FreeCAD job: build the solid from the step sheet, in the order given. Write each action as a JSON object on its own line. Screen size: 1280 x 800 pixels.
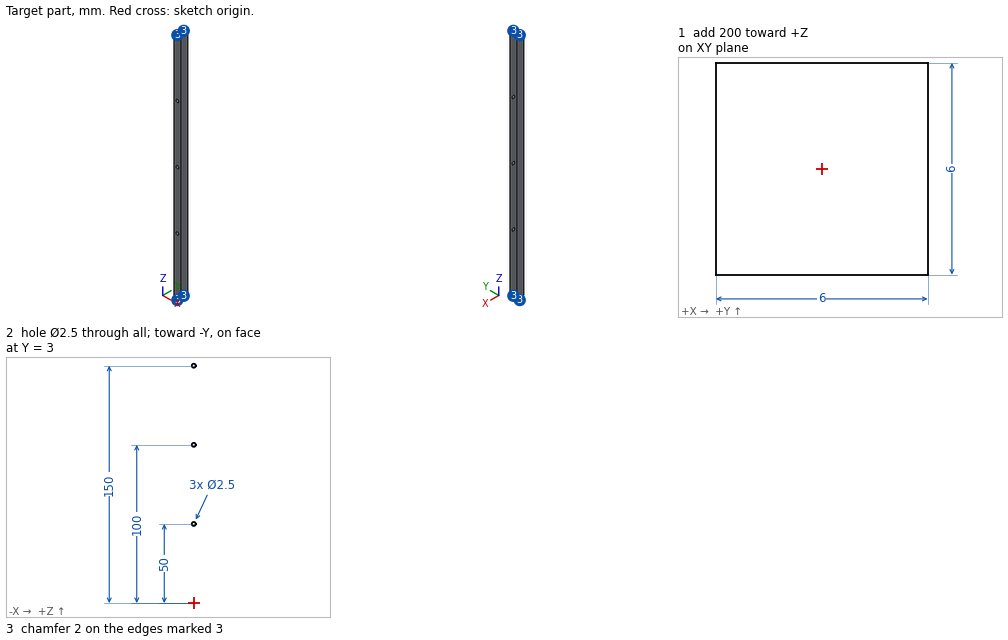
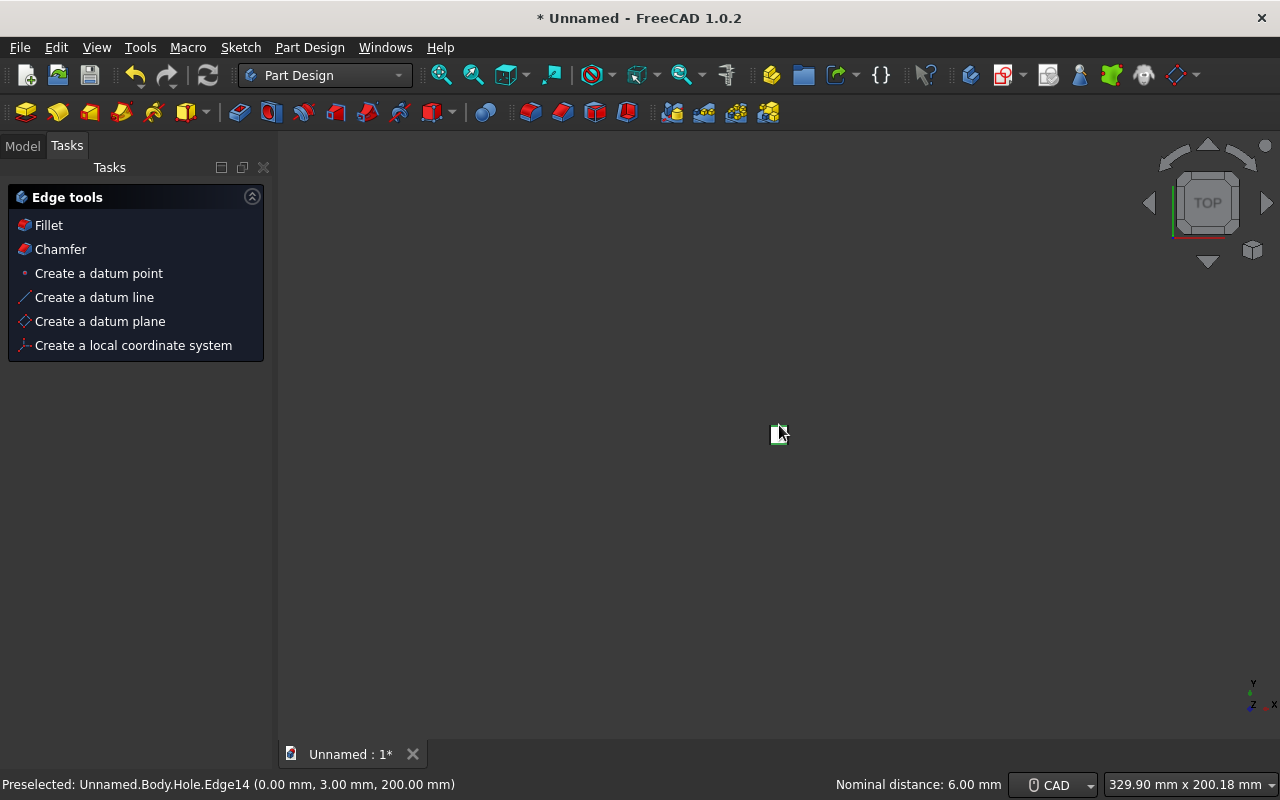
{"action": "scroll", "coordinate": [779, 443], "scroll_direction": "up", "scroll_amount": 4}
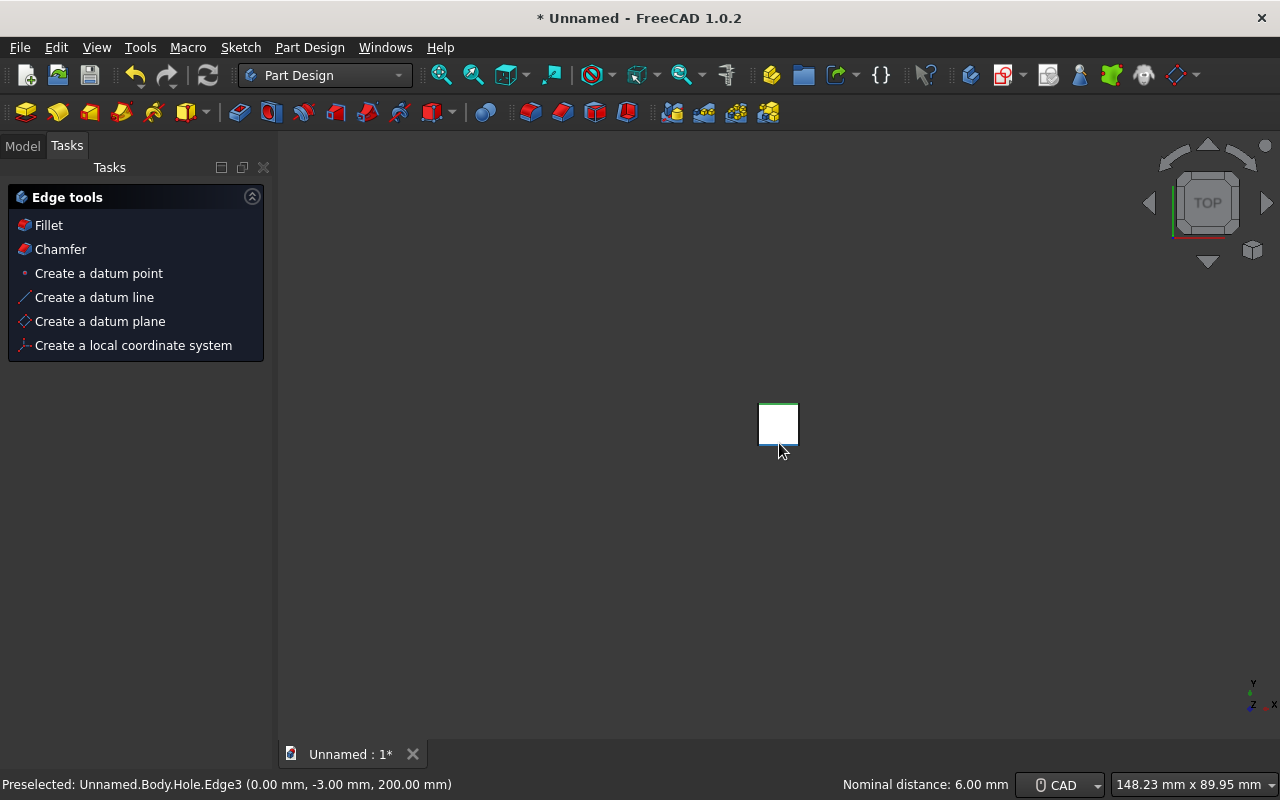
{"action": "left_click", "coordinate": [442, 76]}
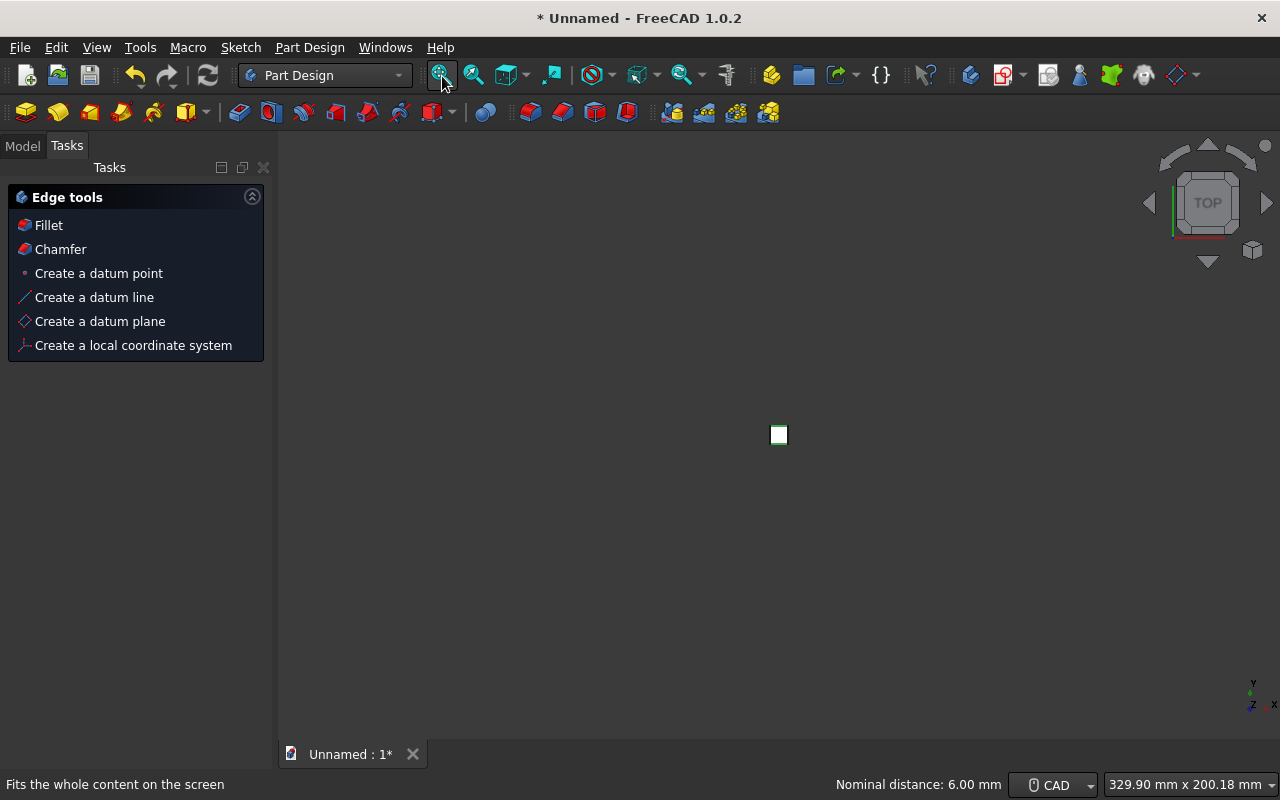
{"action": "key", "text": "1"}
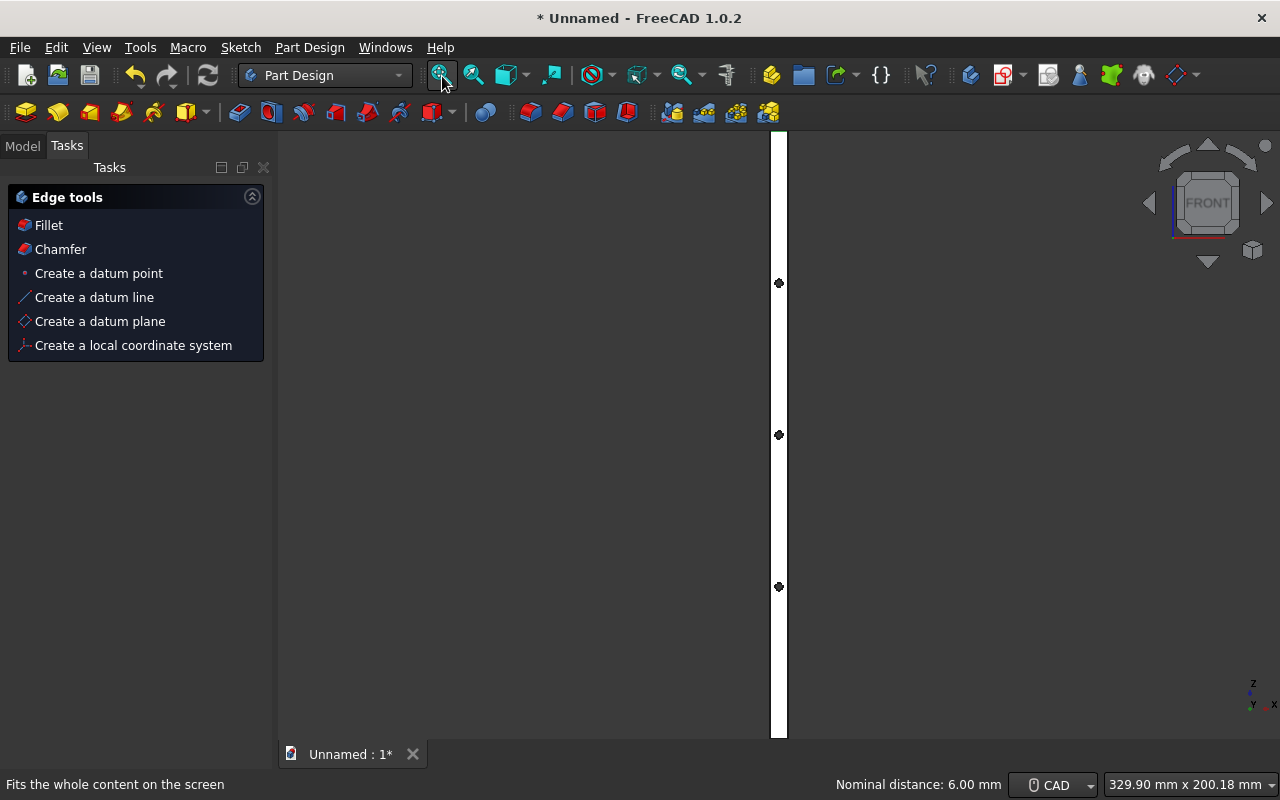
{"action": "left_click", "coordinate": [442, 76]}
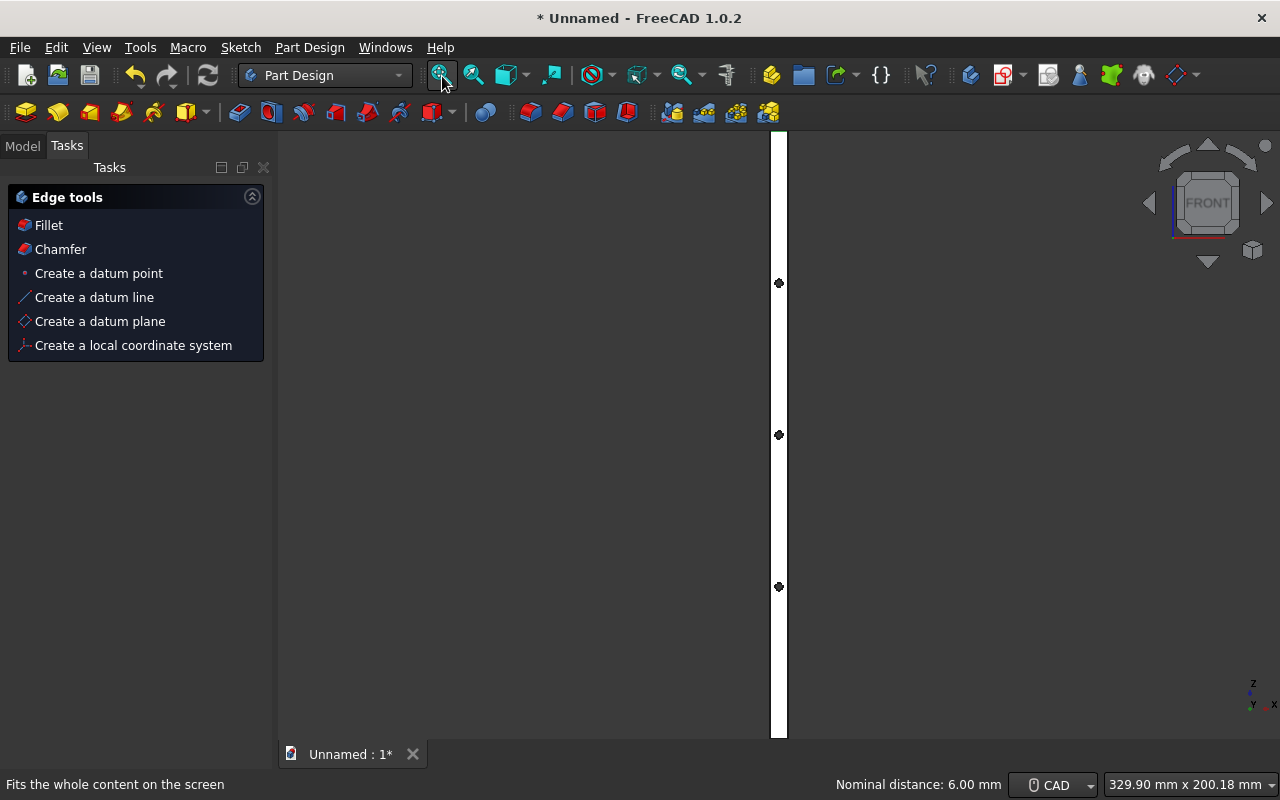
{"action": "key", "text": "3"}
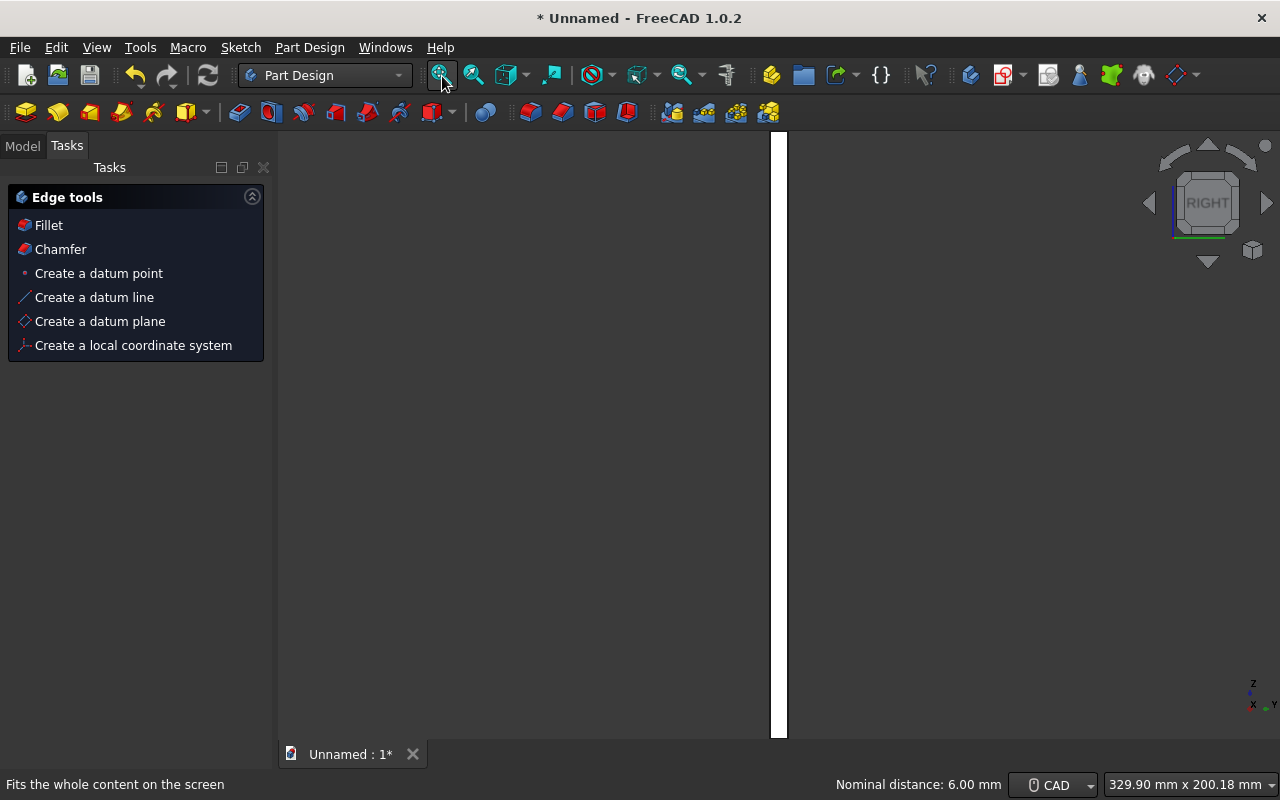
{"action": "left_click", "coordinate": [442, 76]}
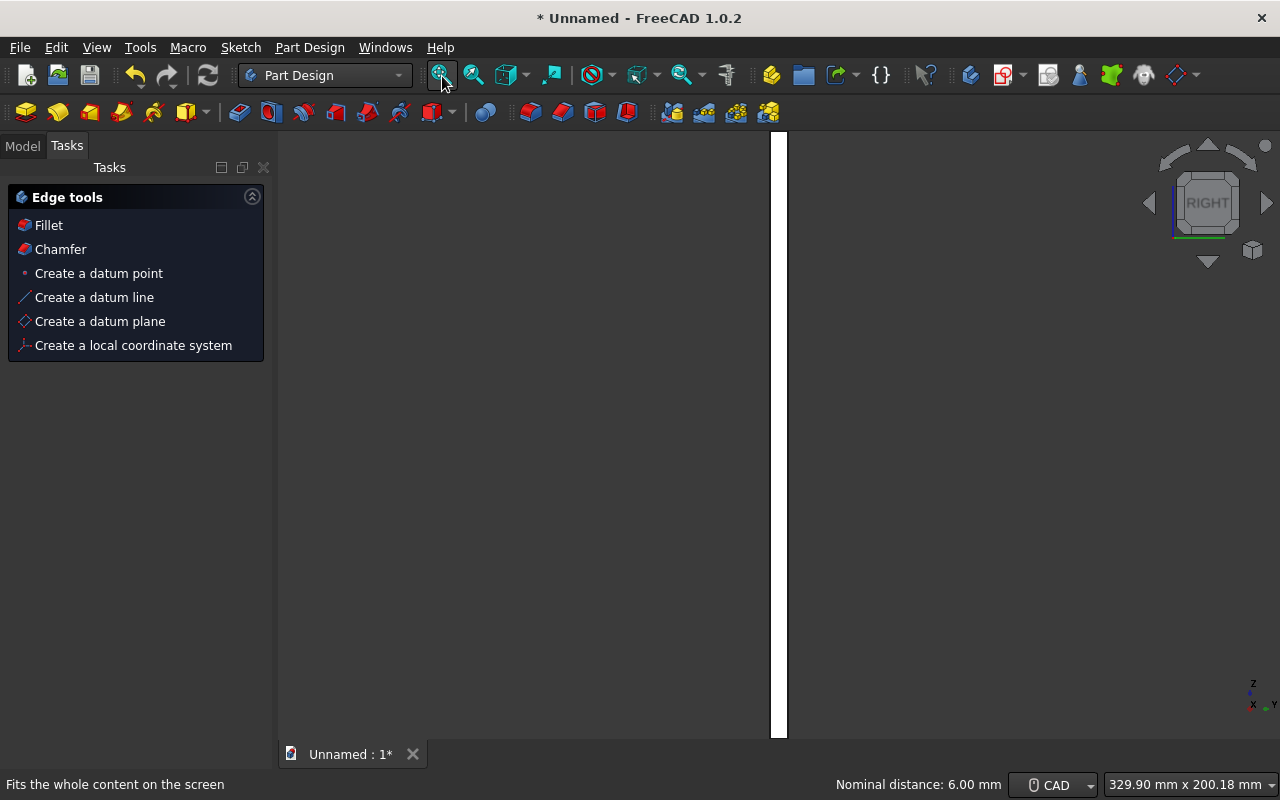
{"action": "key", "text": "5"}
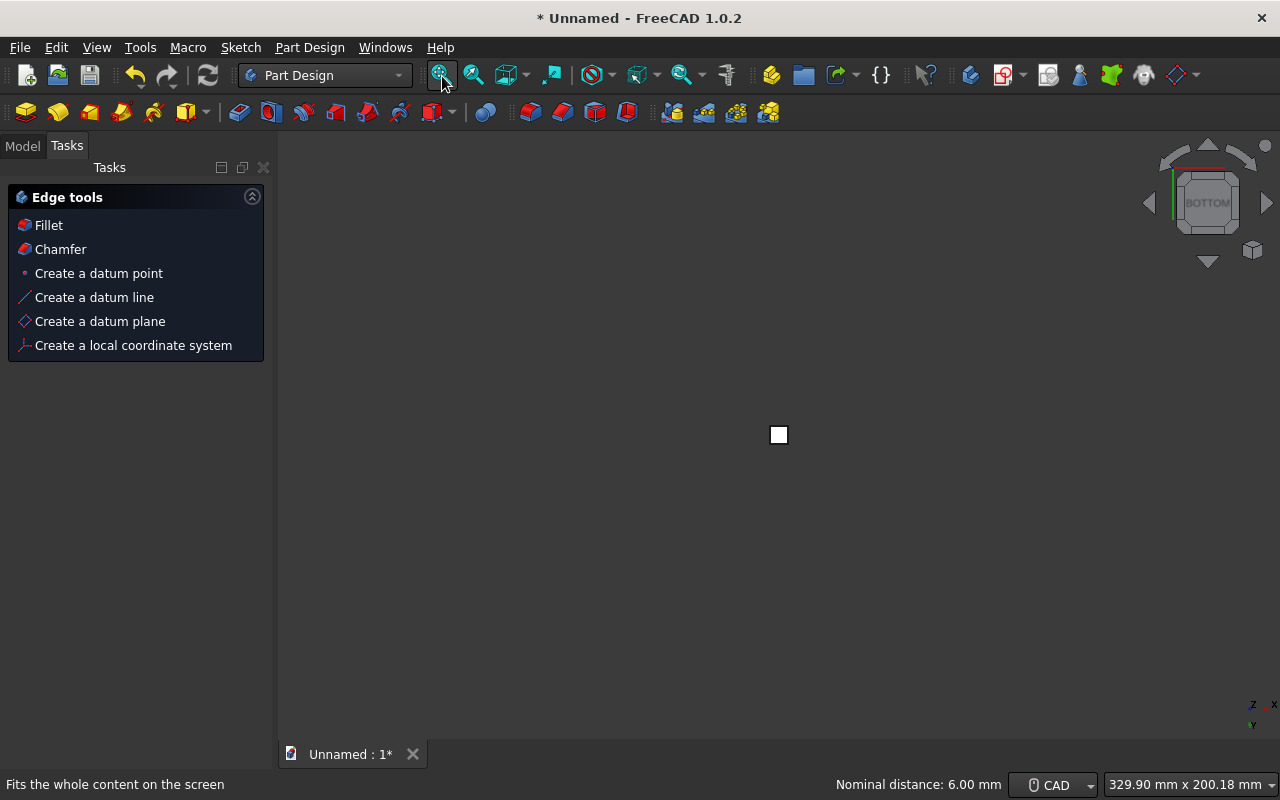
{"action": "left_click", "coordinate": [442, 76]}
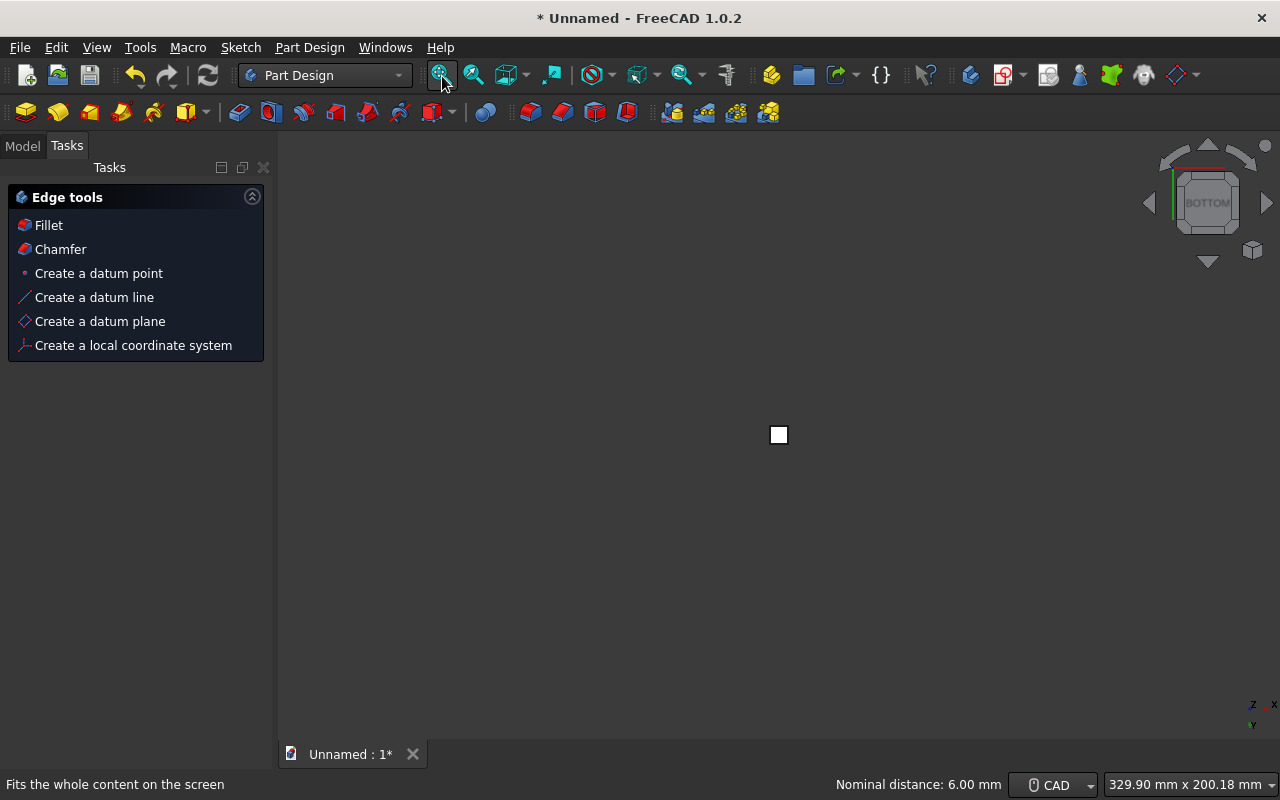
{"action": "left_click", "coordinate": [779, 425], "text": "ctrl"}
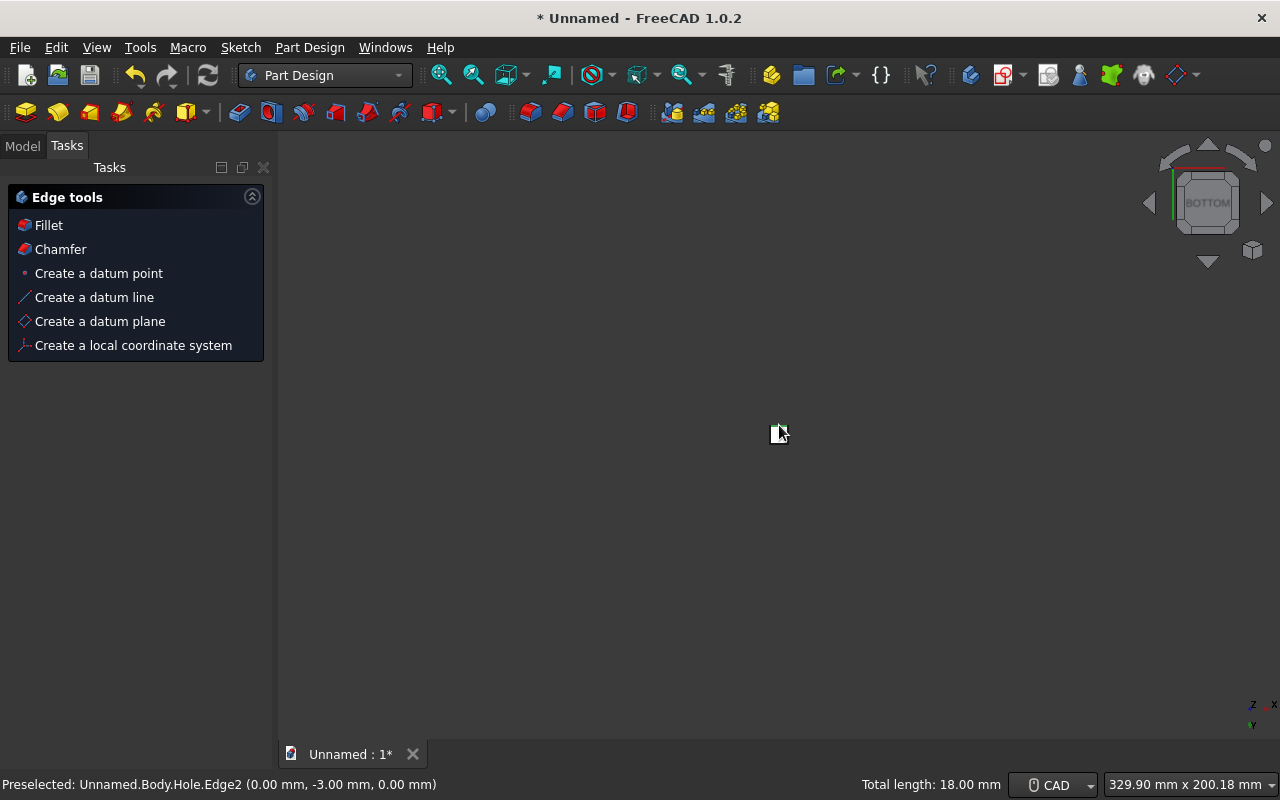
{"action": "left_click", "coordinate": [779, 443], "text": "ctrl"}